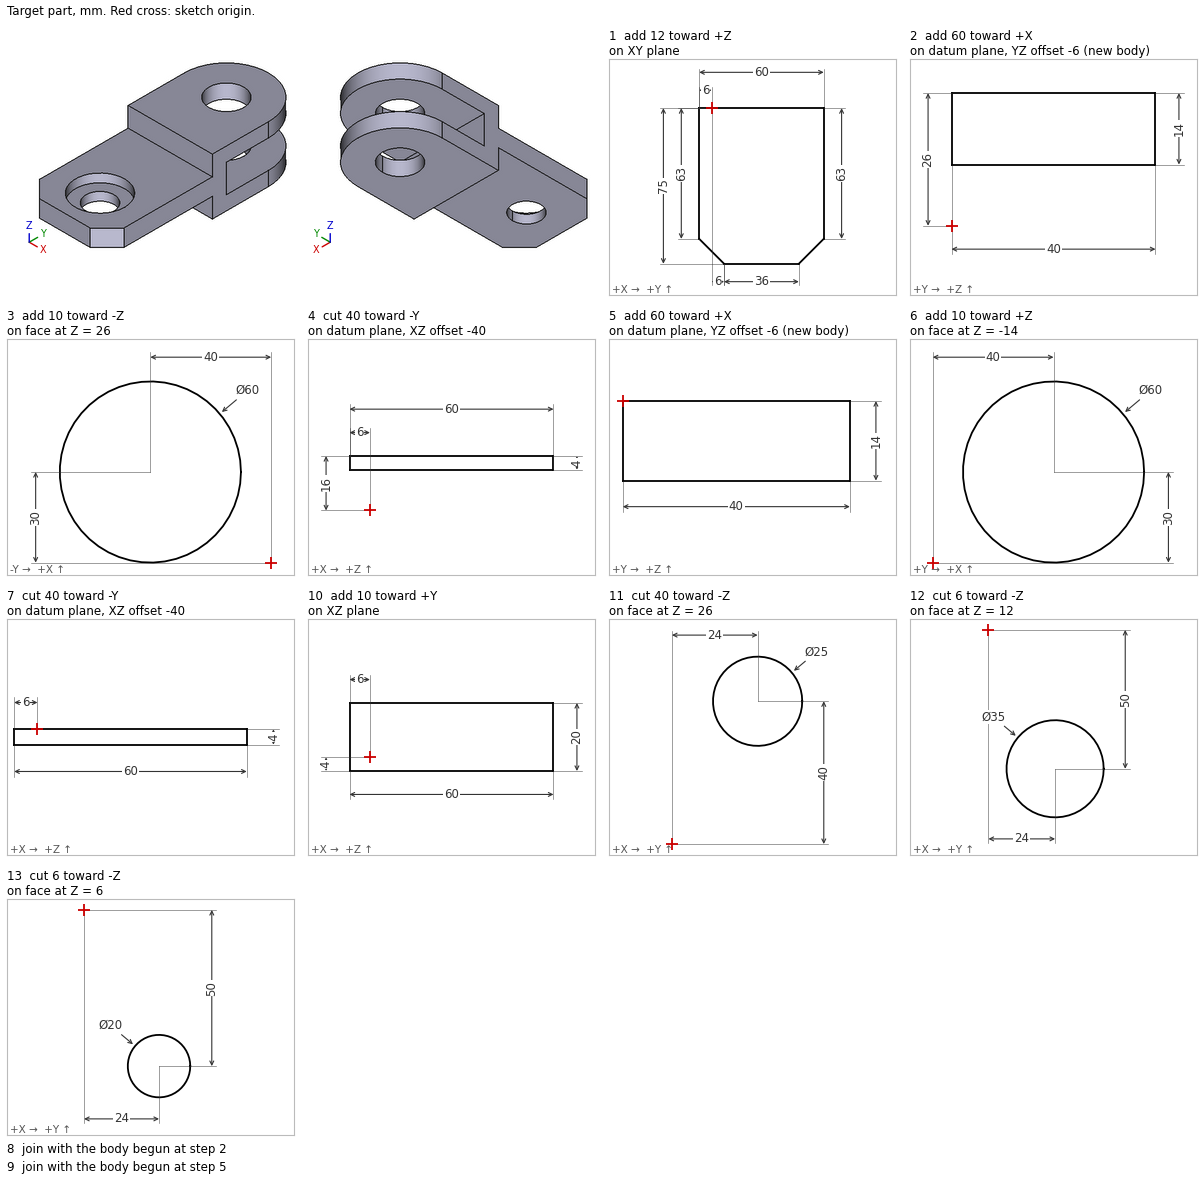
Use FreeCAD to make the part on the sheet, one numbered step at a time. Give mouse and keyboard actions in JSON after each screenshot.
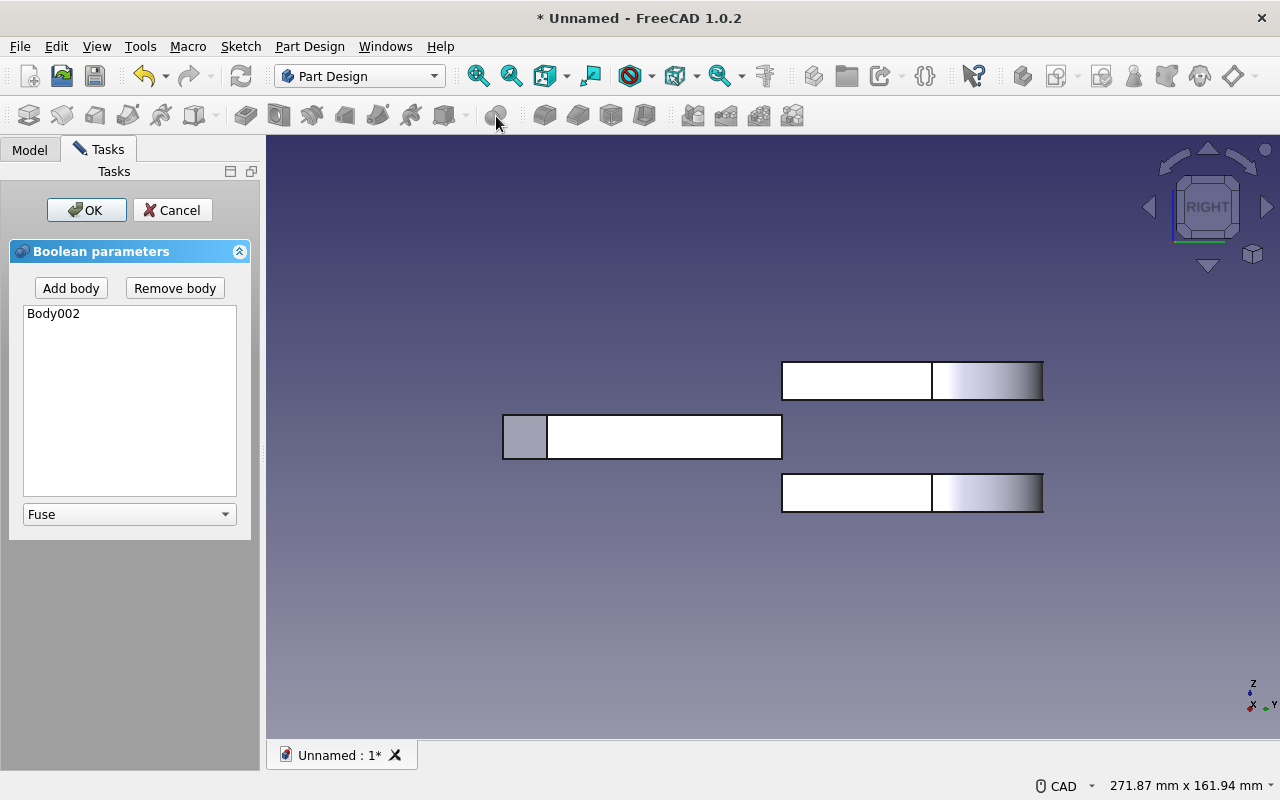
{"action": "left_click", "coordinate": [87, 210]}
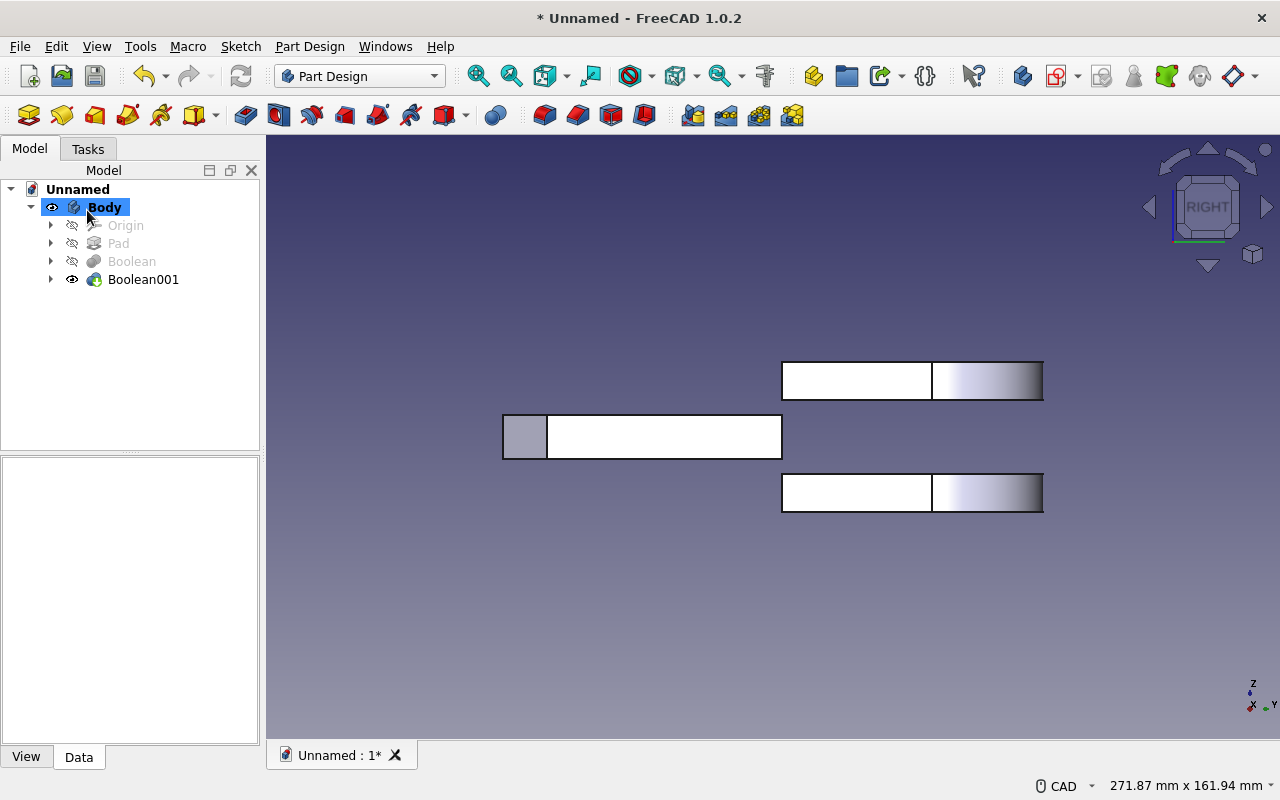
{"action": "left_click", "coordinate": [1056, 76]}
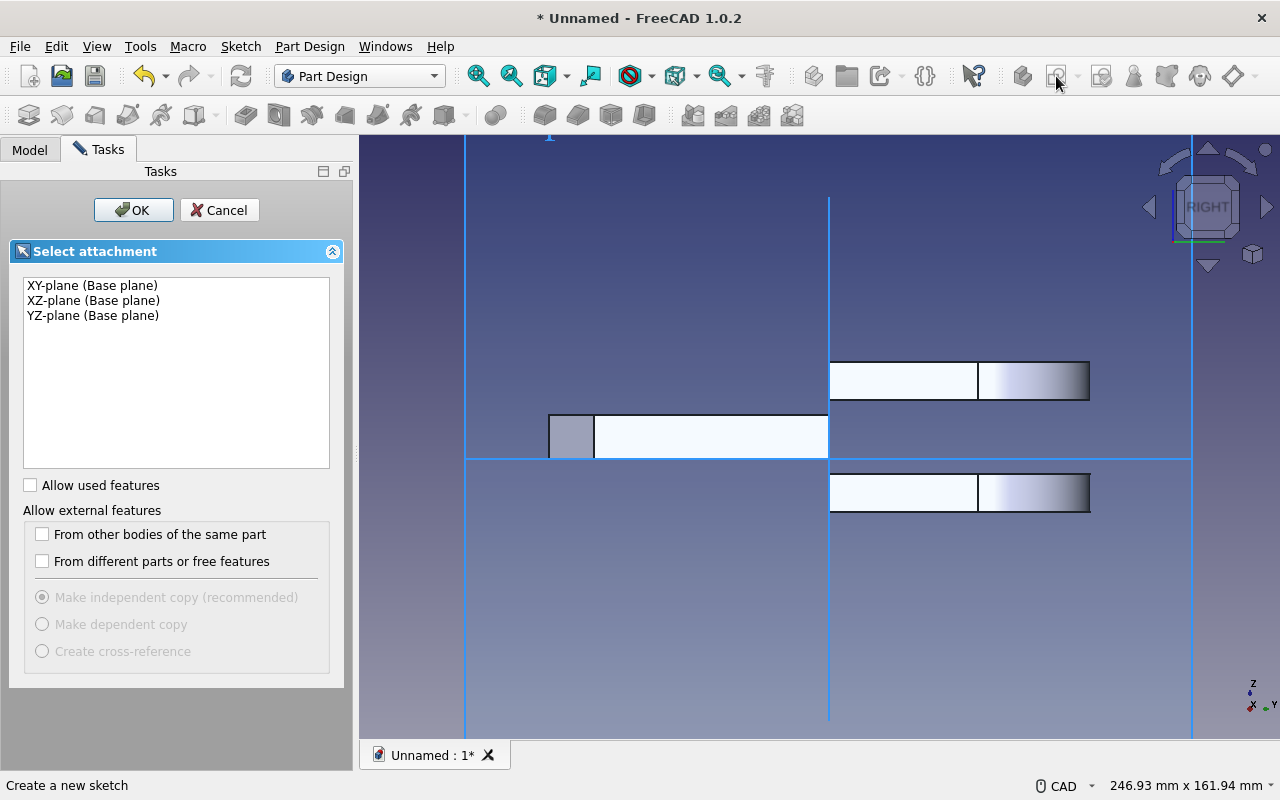
{"action": "left_click", "coordinate": [84, 300]}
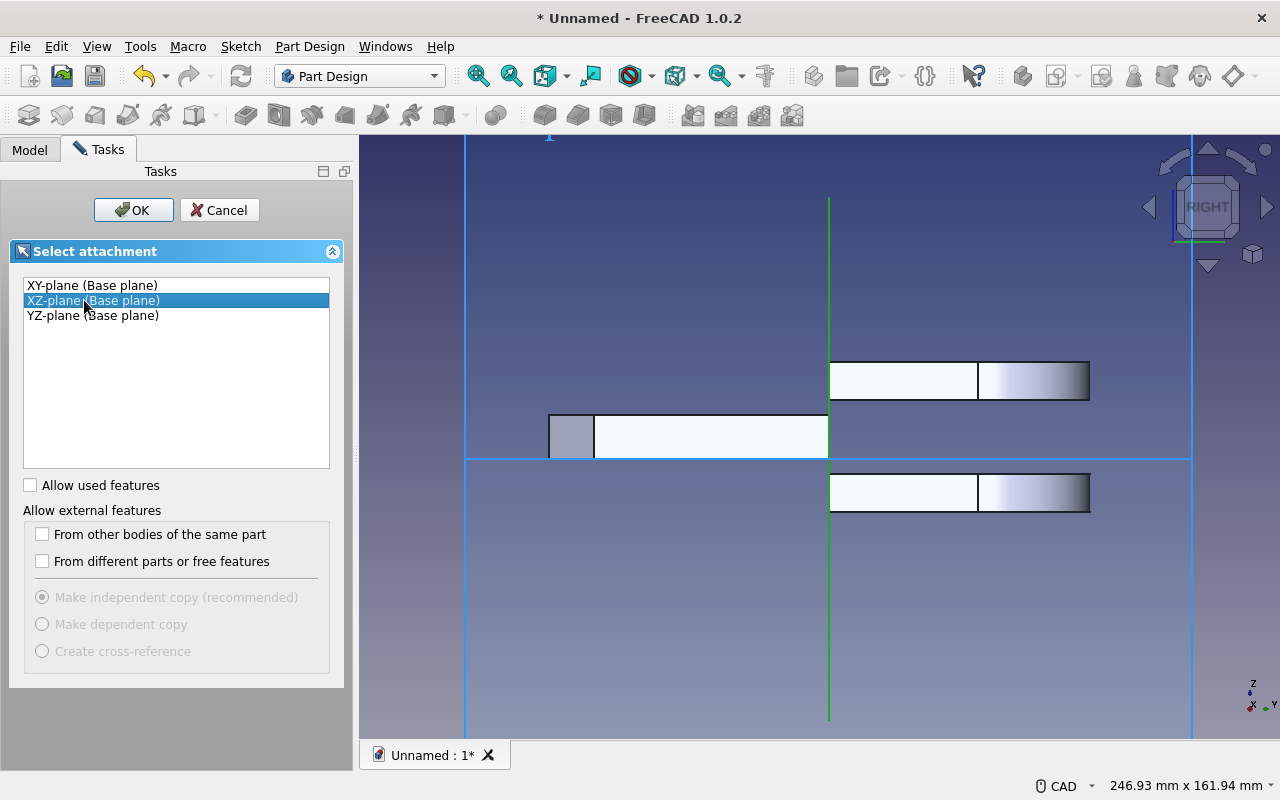
{"action": "left_click", "coordinate": [134, 210]}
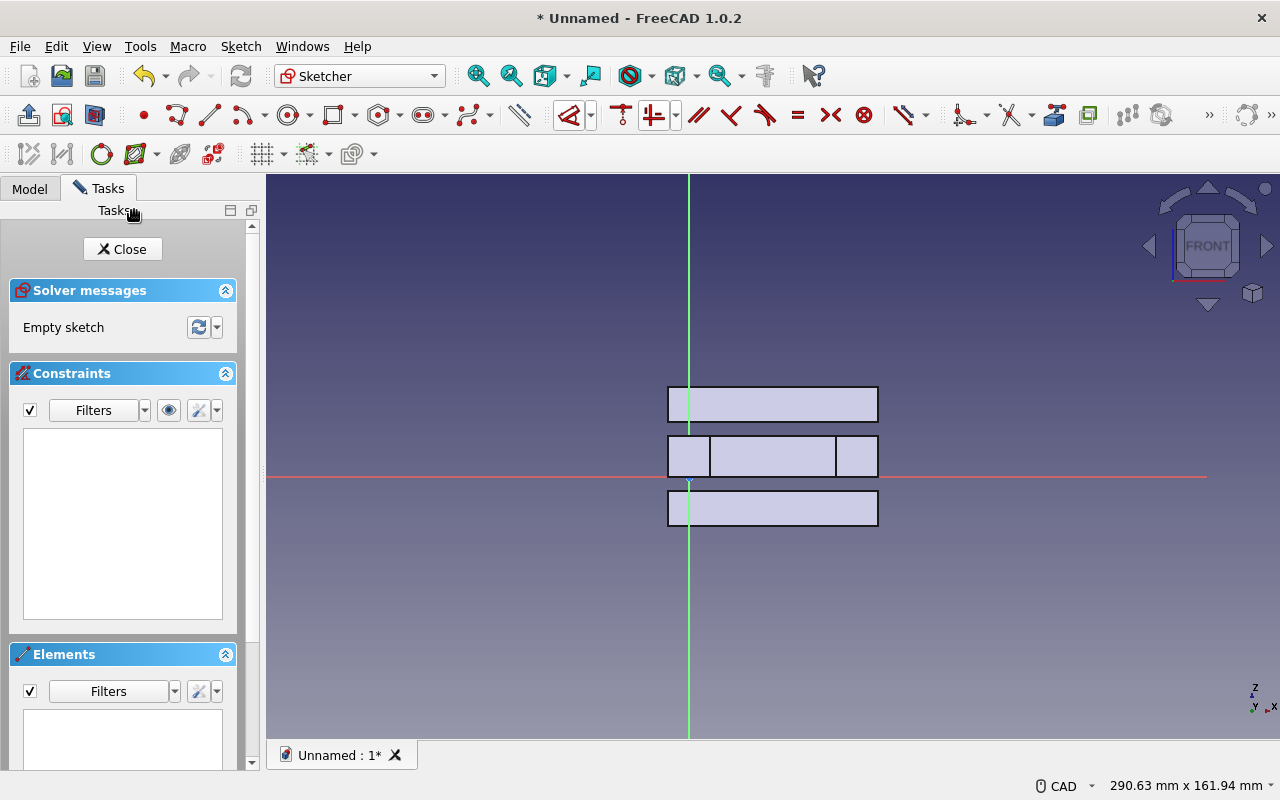
{"action": "left_click", "coordinate": [95, 116]}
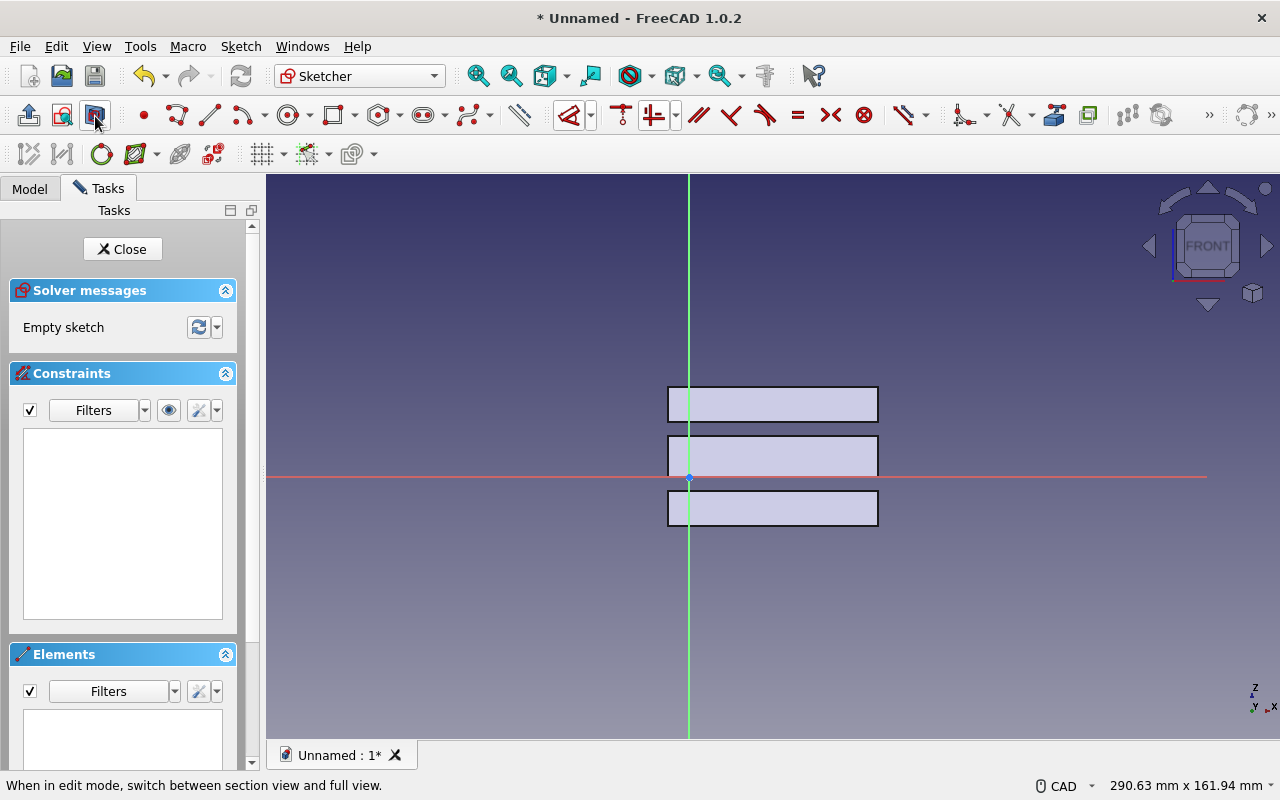
{"action": "scroll", "coordinate": [813, 457], "scroll_direction": "up", "scroll_amount": 5}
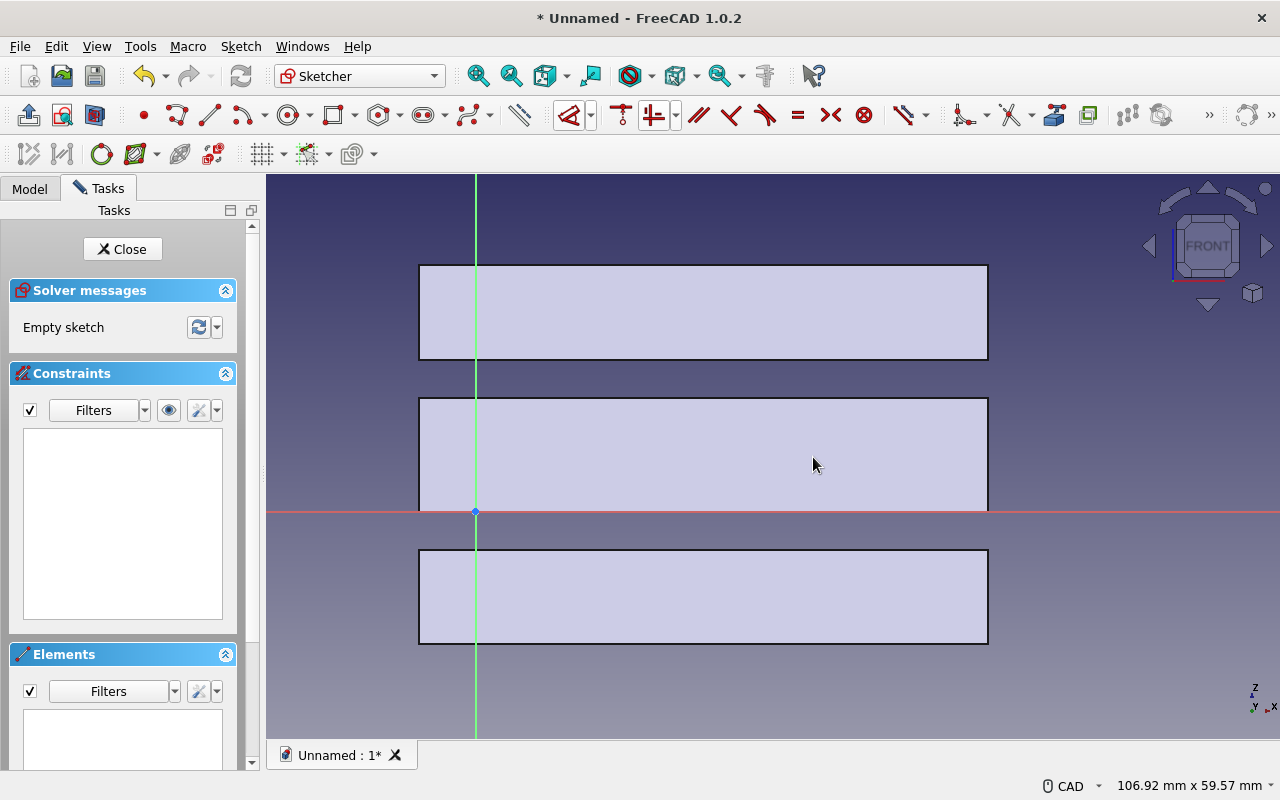
{"action": "left_click", "coordinate": [332, 116]}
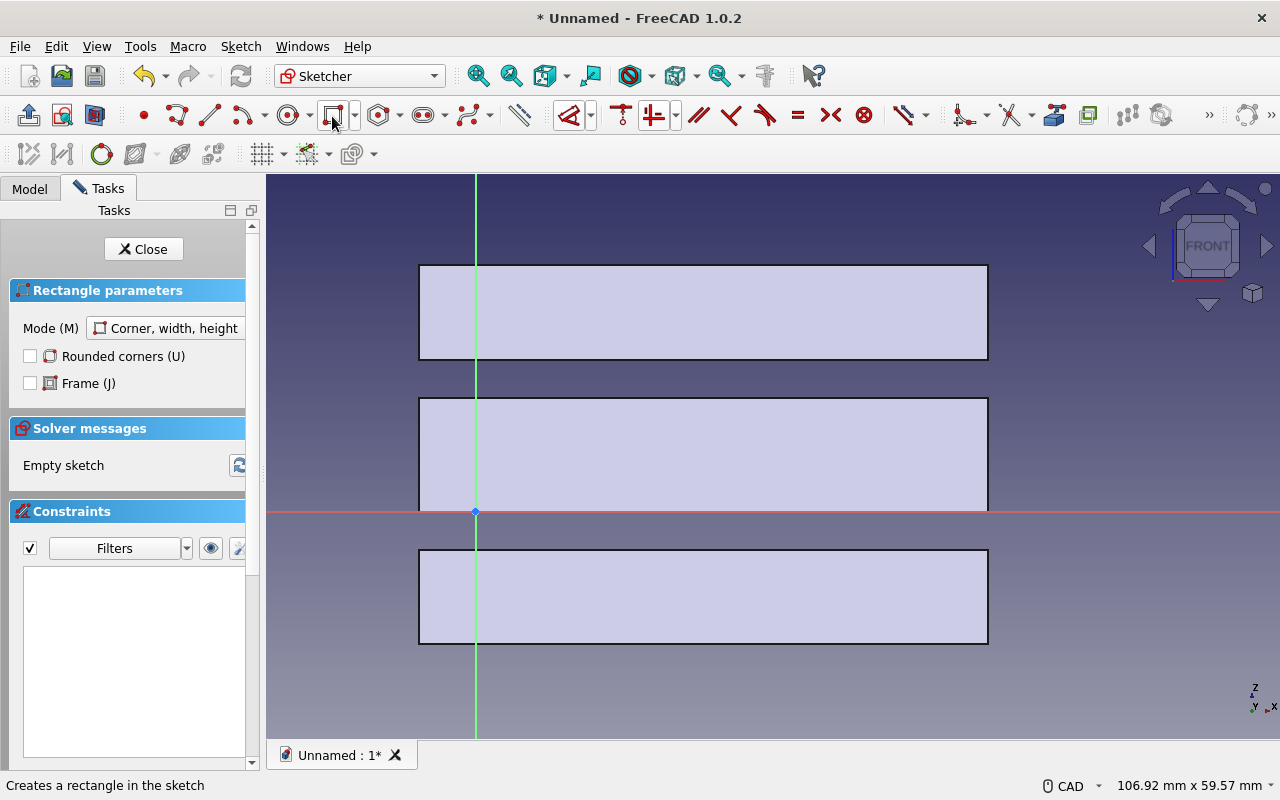
{"action": "left_click", "coordinate": [419, 360]}
{"action": "mouse_move", "coordinate": [988, 550]}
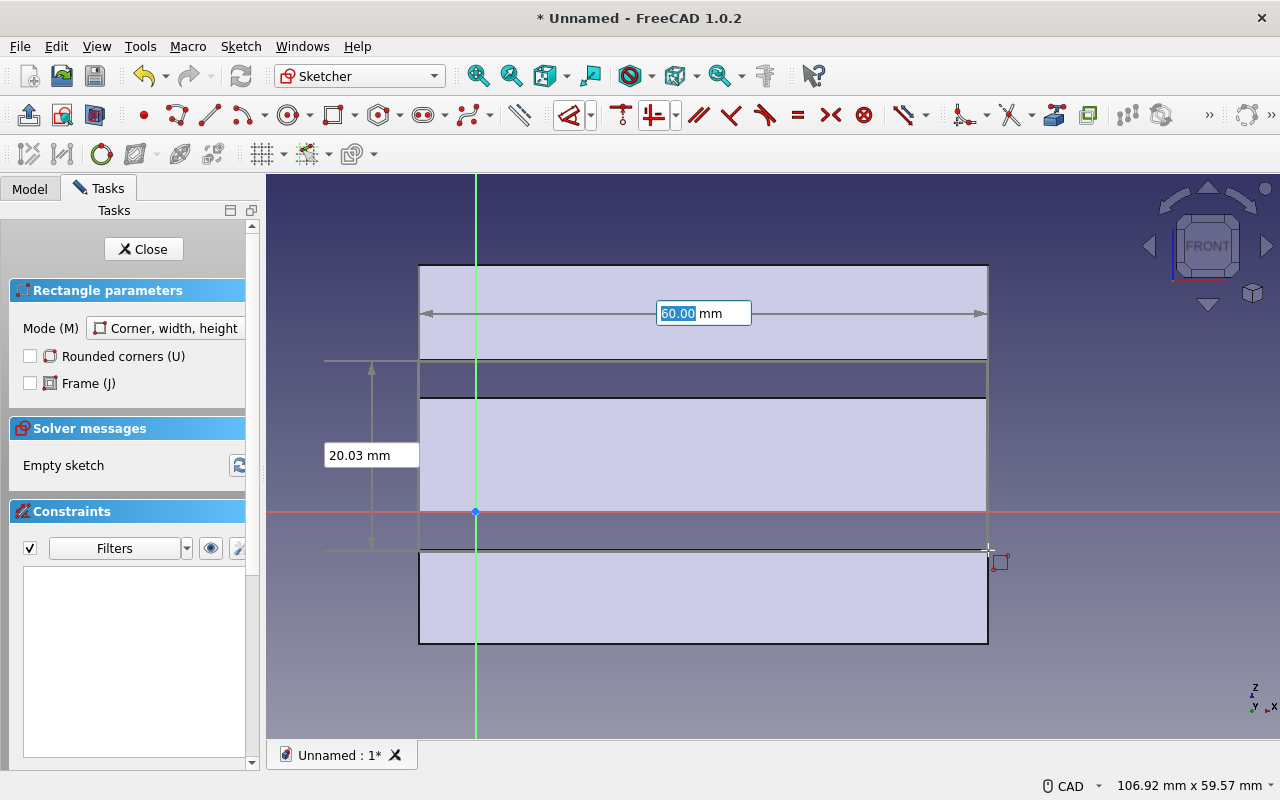
{"action": "type", "text": "60"}
{"action": "key", "text": "Tab"}
{"action": "type", "text": "20"}
{"action": "key", "text": "Return"}
{"action": "key", "text": "Escape"}